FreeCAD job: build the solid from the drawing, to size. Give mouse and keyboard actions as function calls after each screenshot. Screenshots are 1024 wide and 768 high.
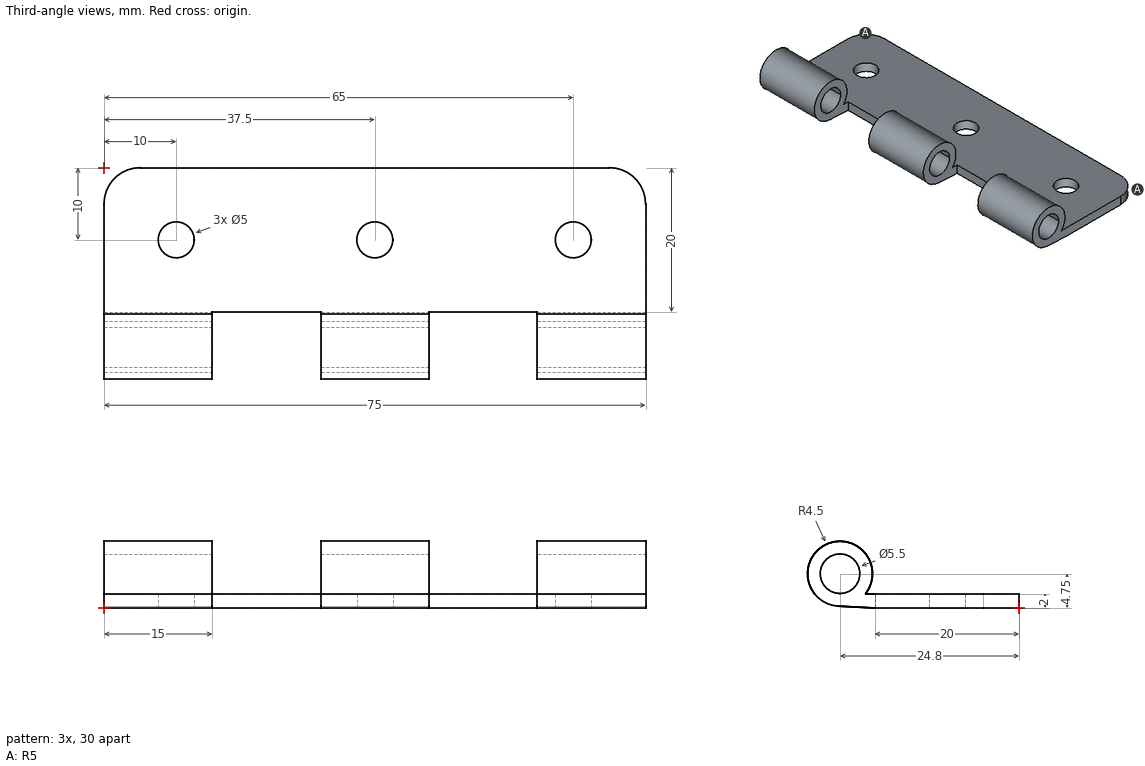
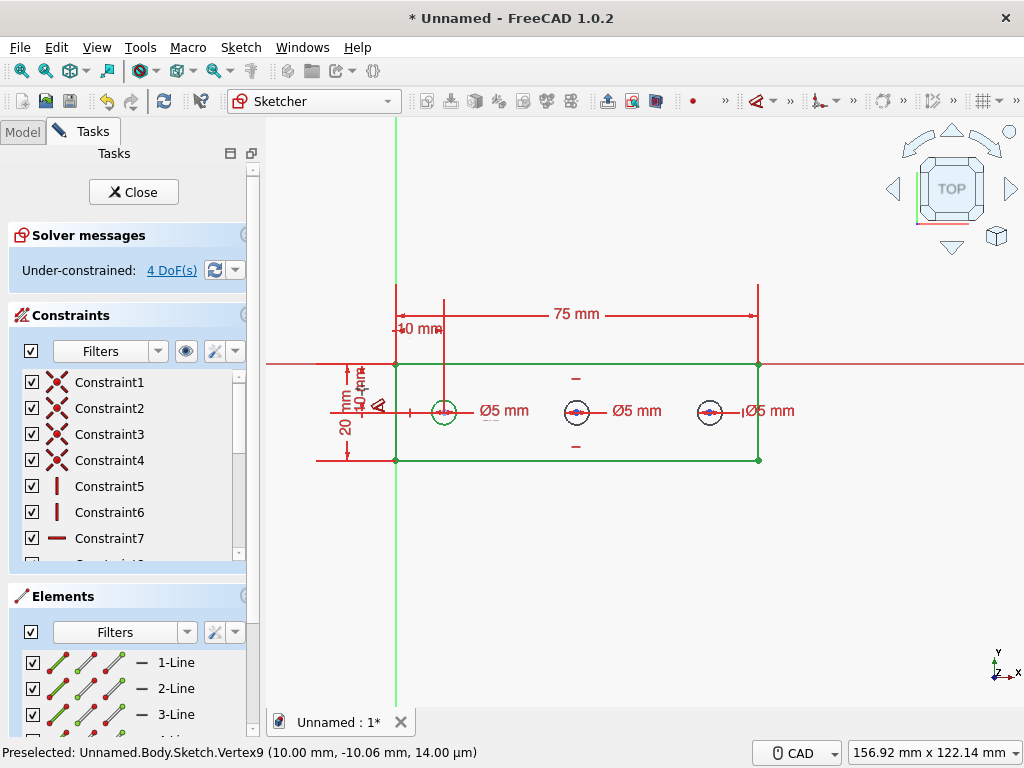
click(577, 413)
click(611, 389)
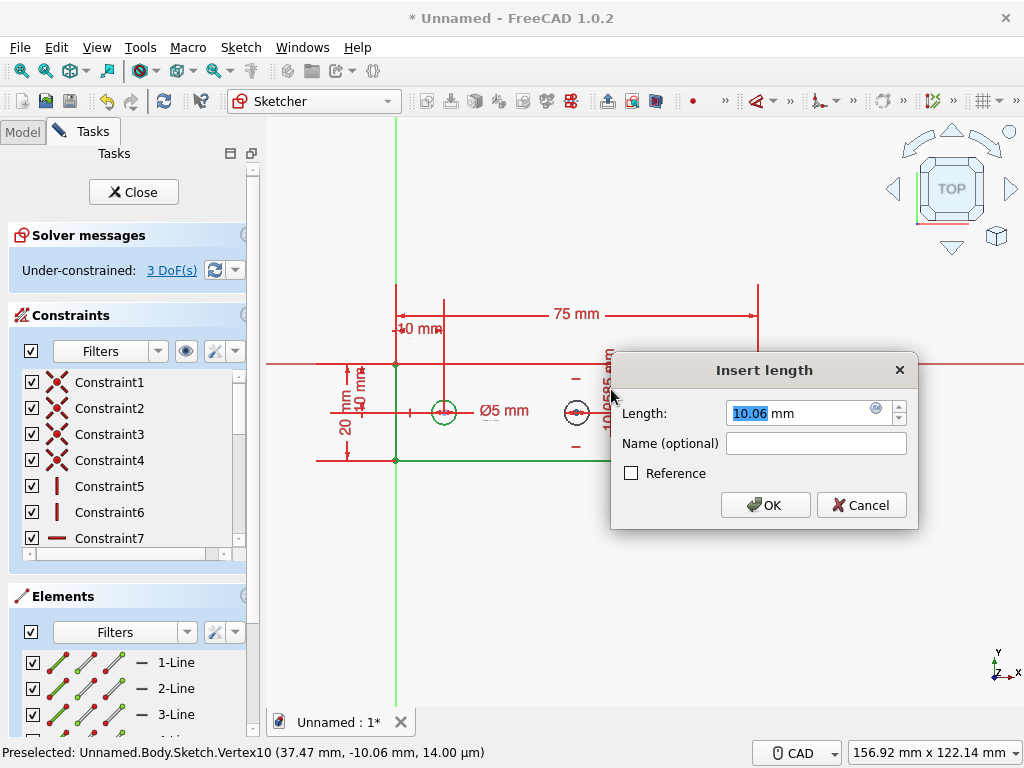
text(10)
key(Return)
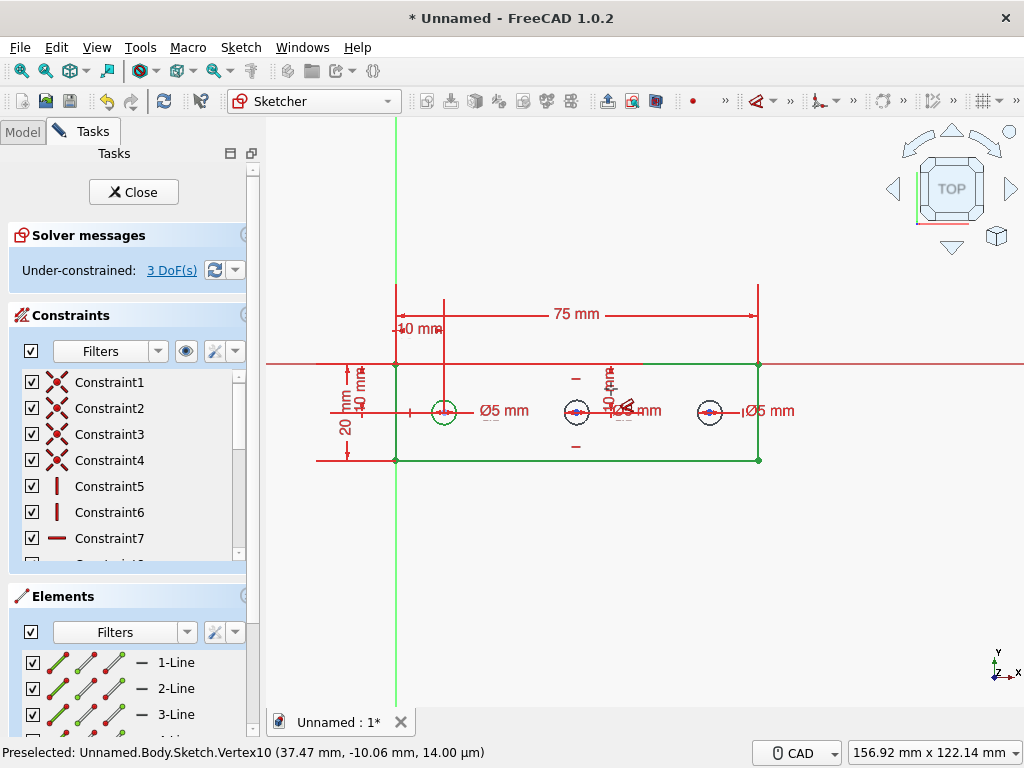
click(710, 413)
click(553, 330)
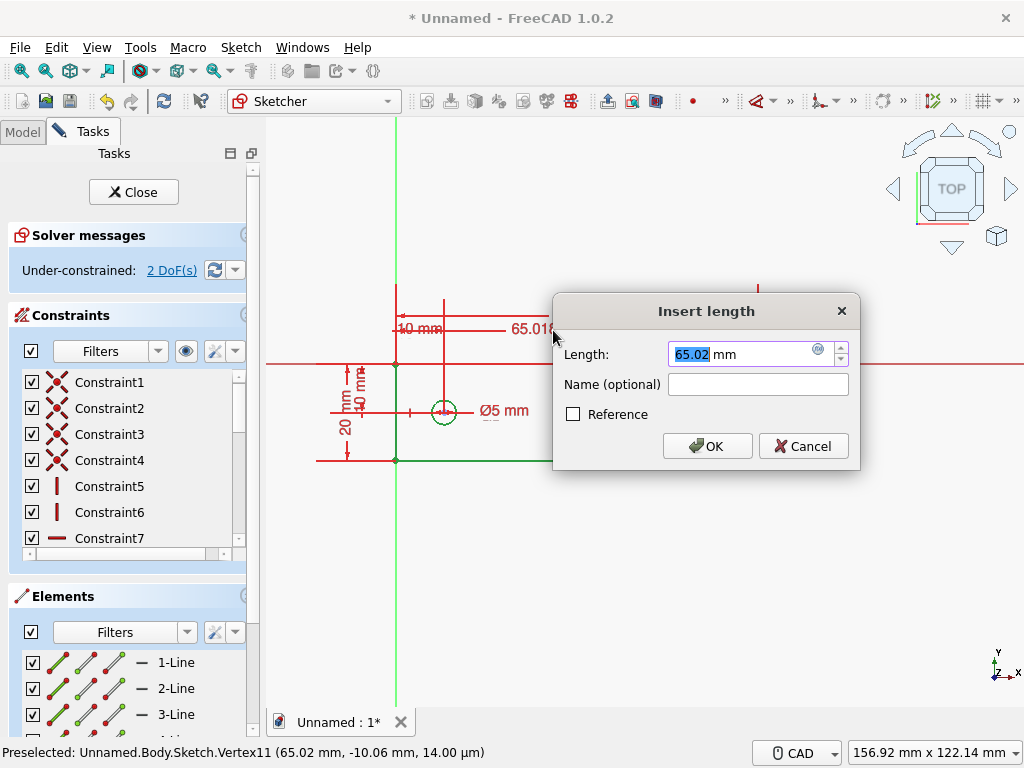
text(65)
key(Return)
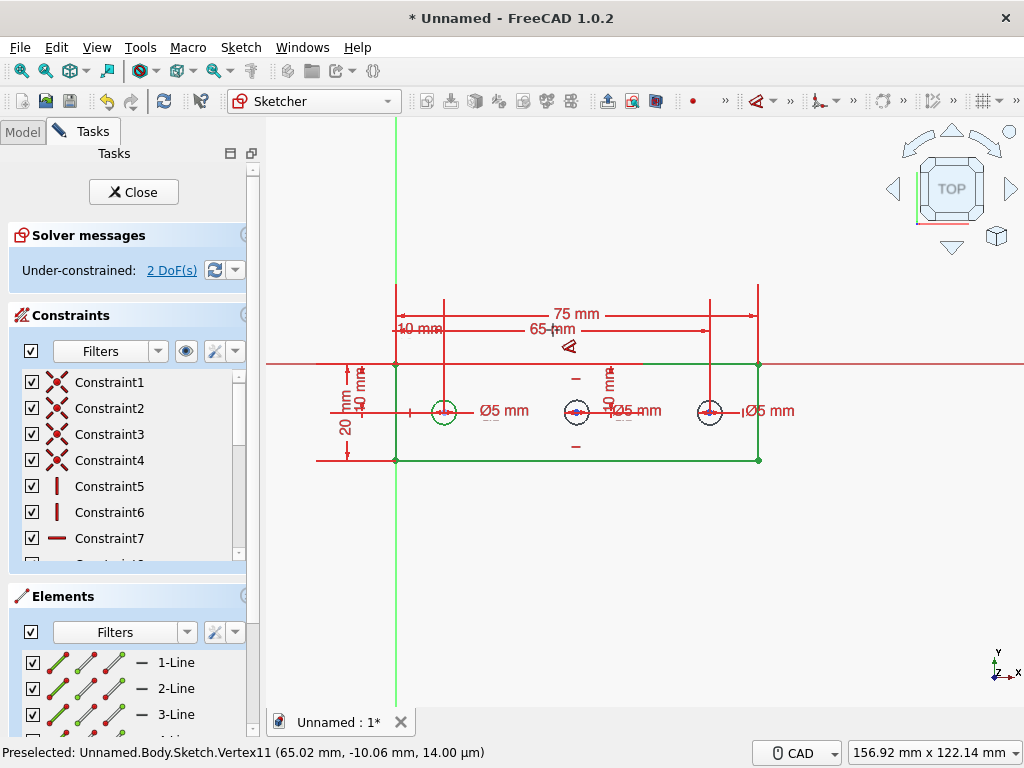
click(710, 413)
click(744, 389)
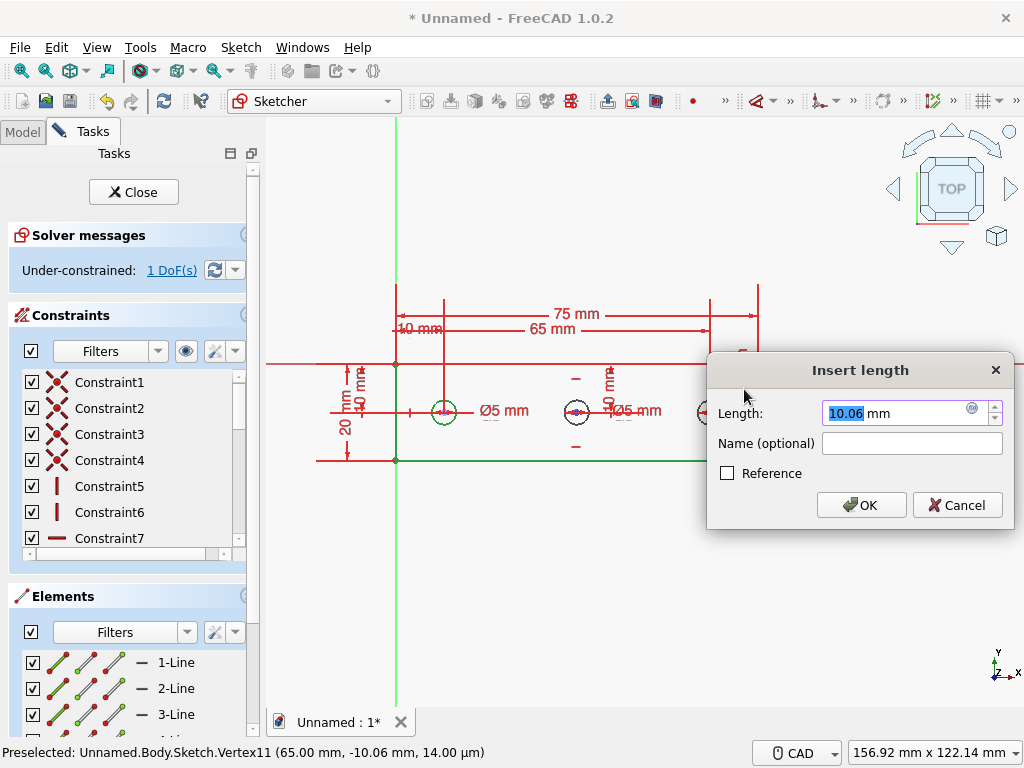
text(10)
key(Return)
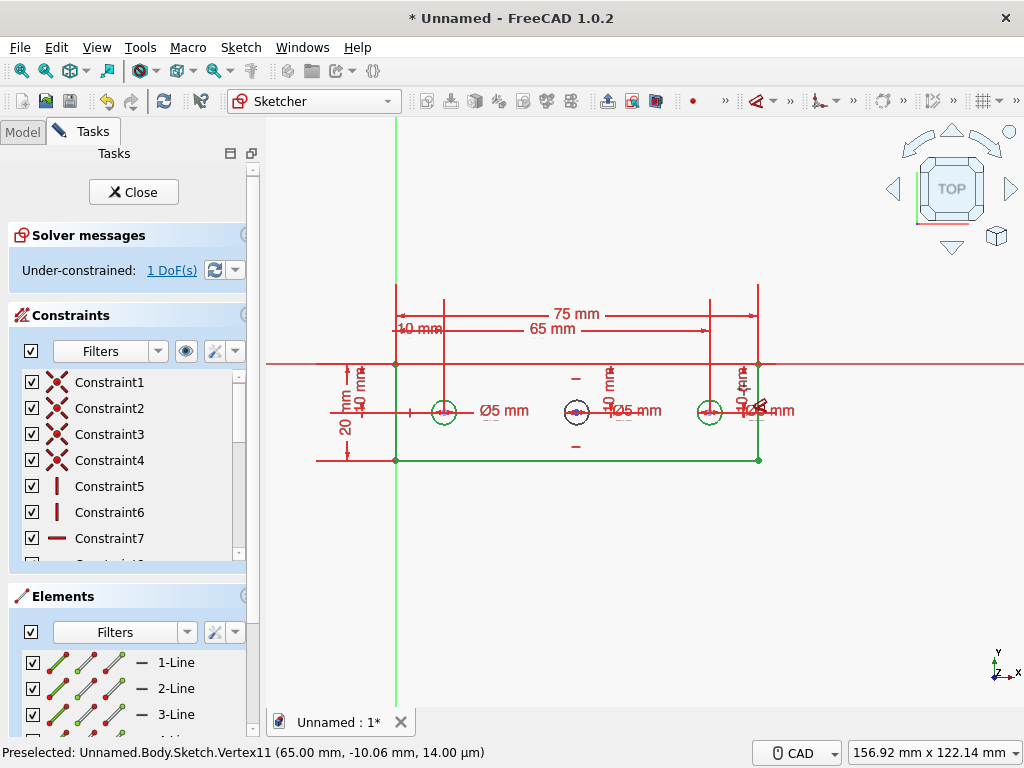
click(577, 413)
click(486, 447)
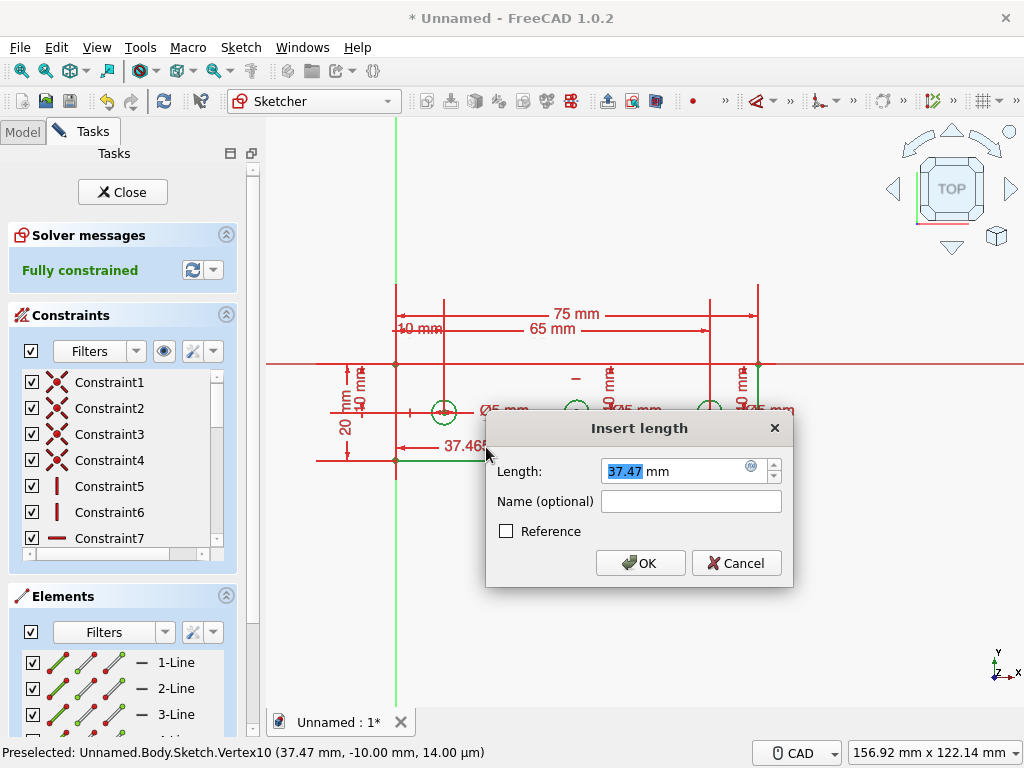
text(37.5)
key(Return)
key(Escape)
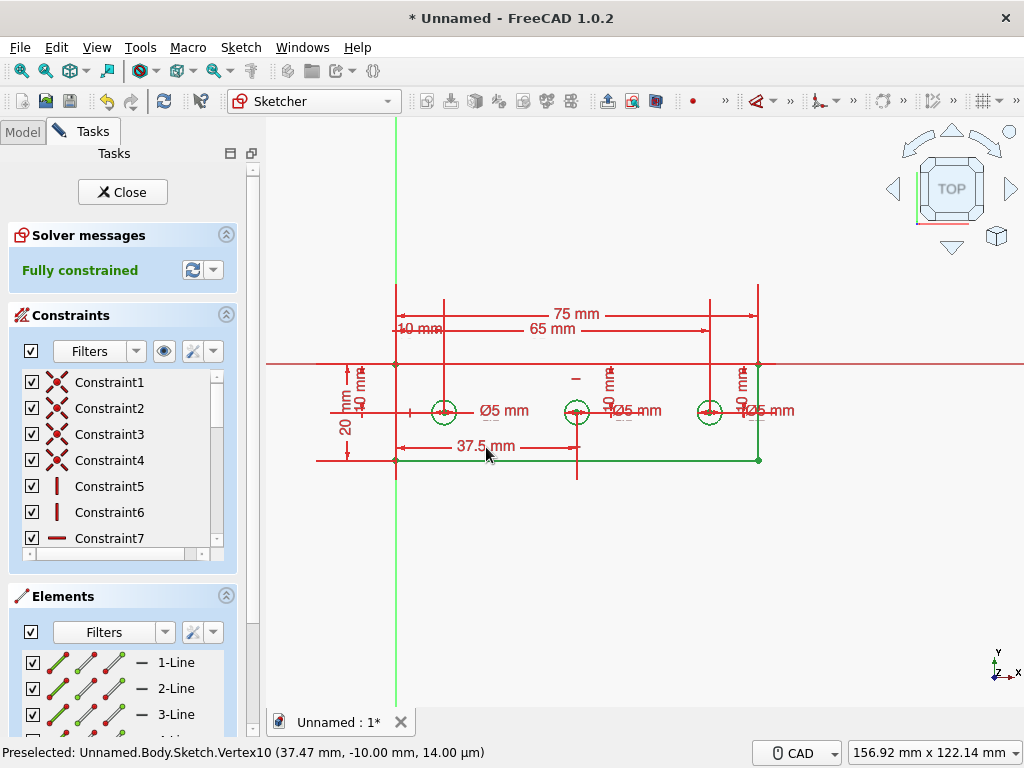
click(123, 192)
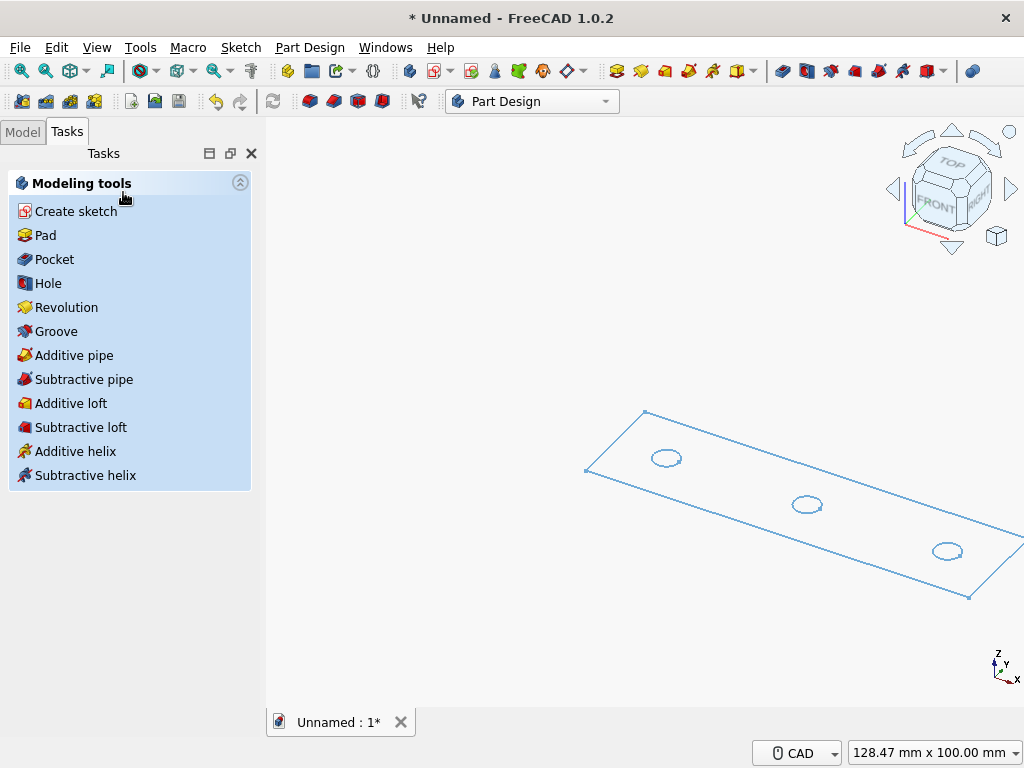
click(618, 72)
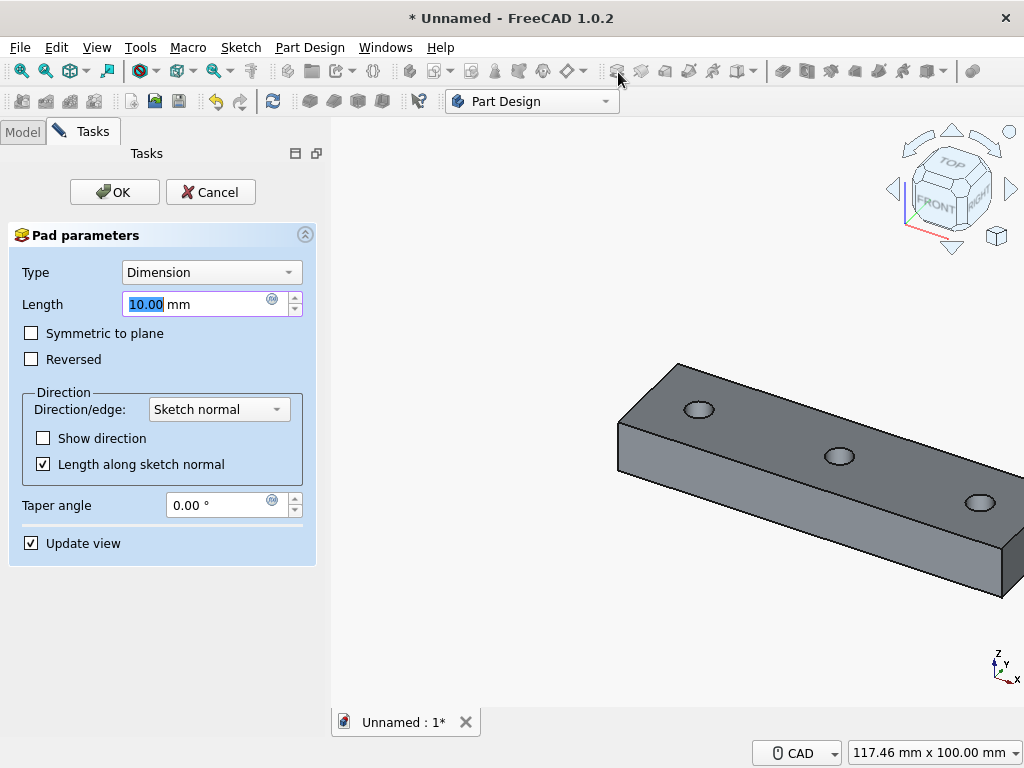
text(2)
key(Tab)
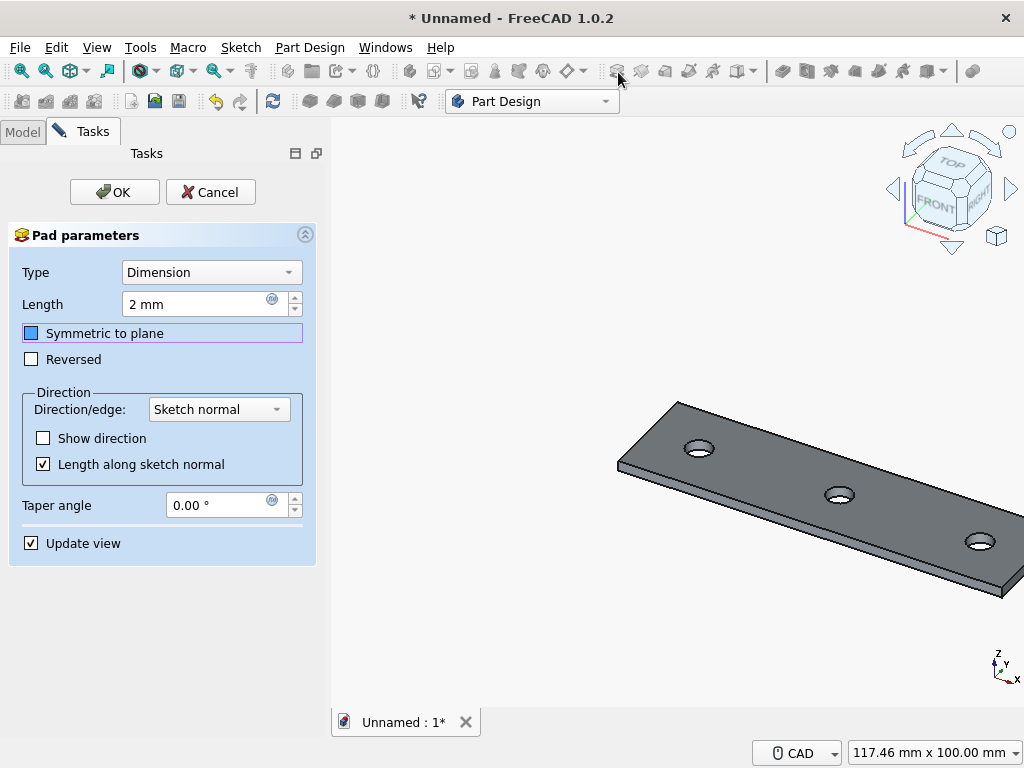
click(115, 192)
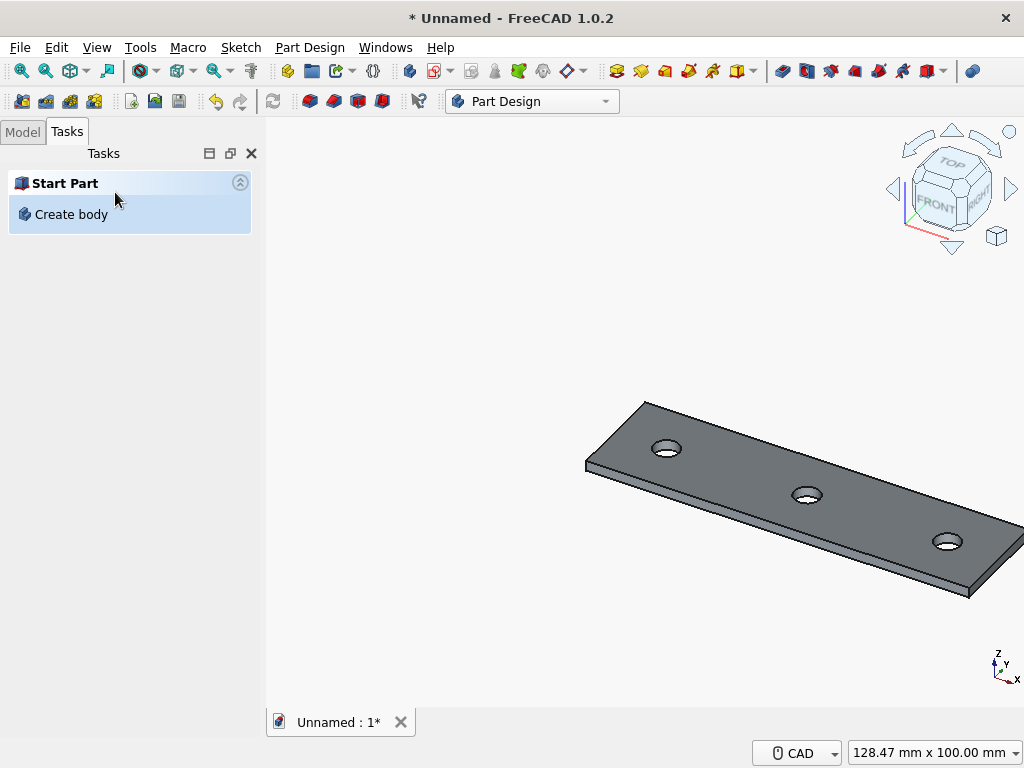
click(22, 72)